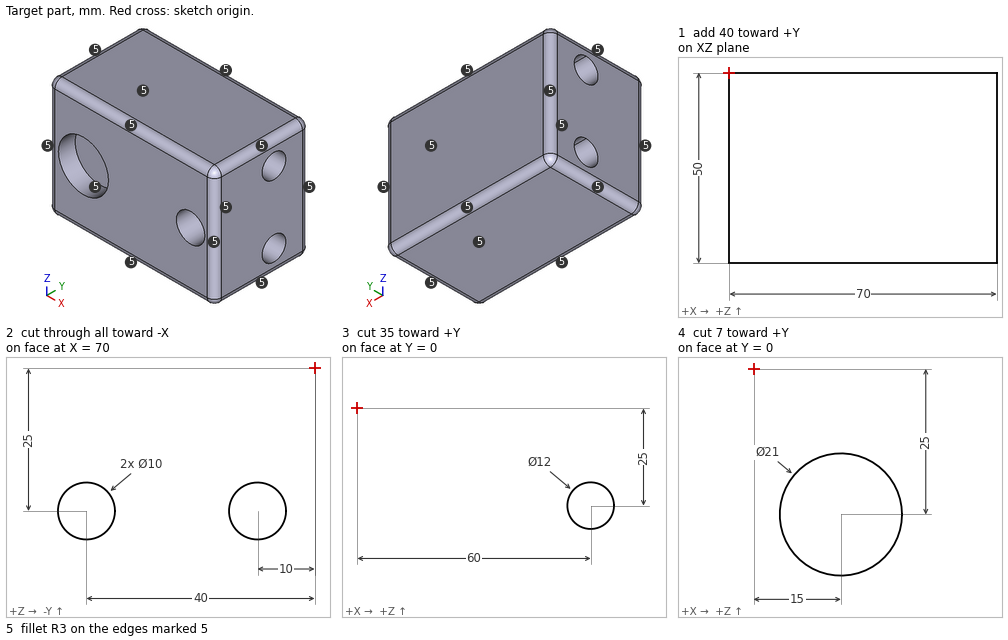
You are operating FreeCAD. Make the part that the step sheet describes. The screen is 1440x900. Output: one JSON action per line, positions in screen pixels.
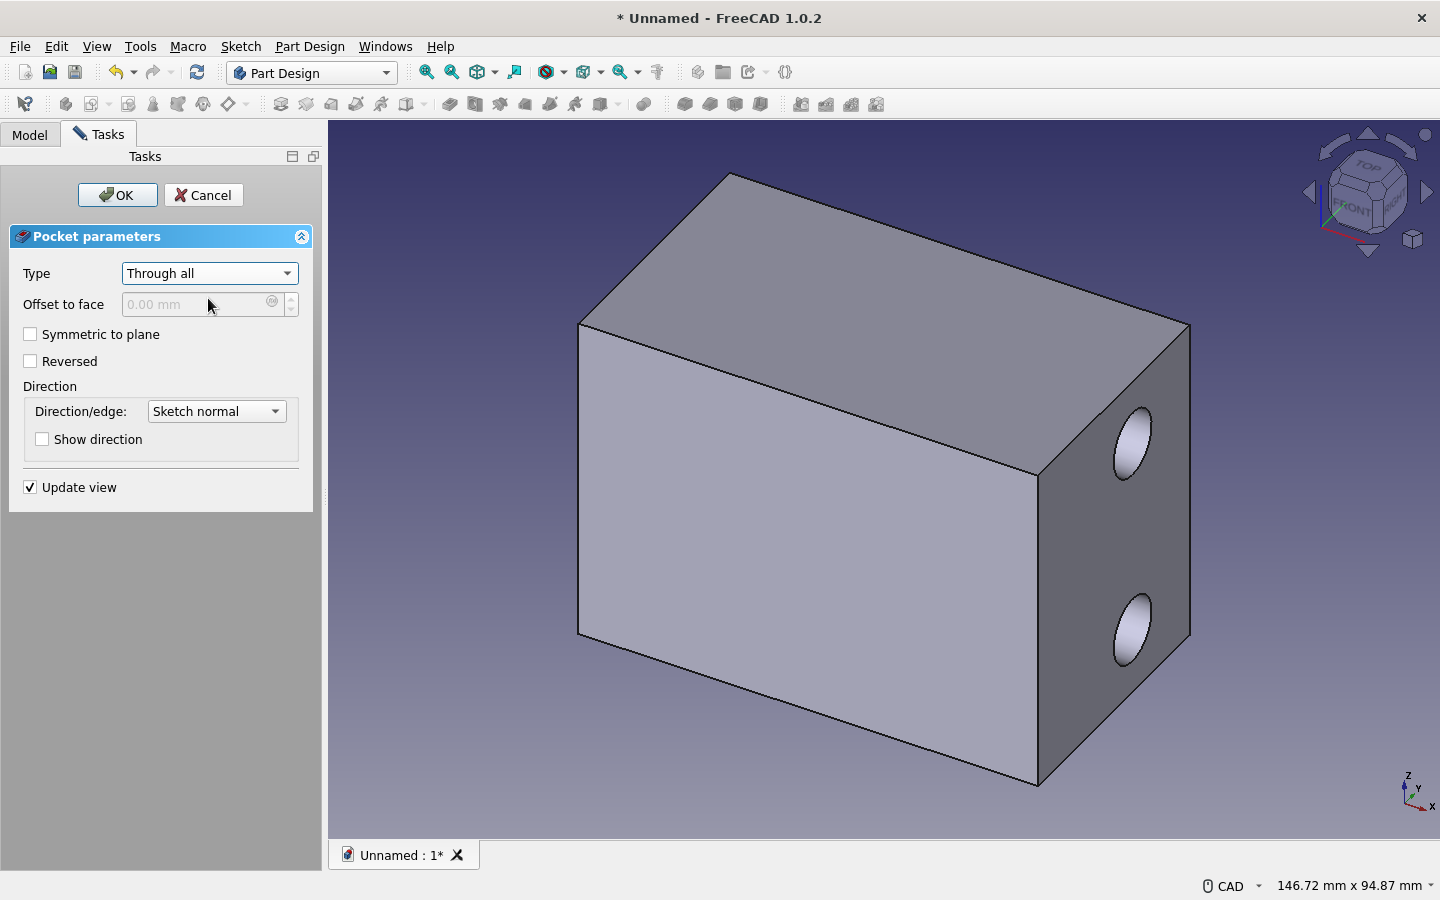
{"action": "left_click", "coordinate": [118, 195]}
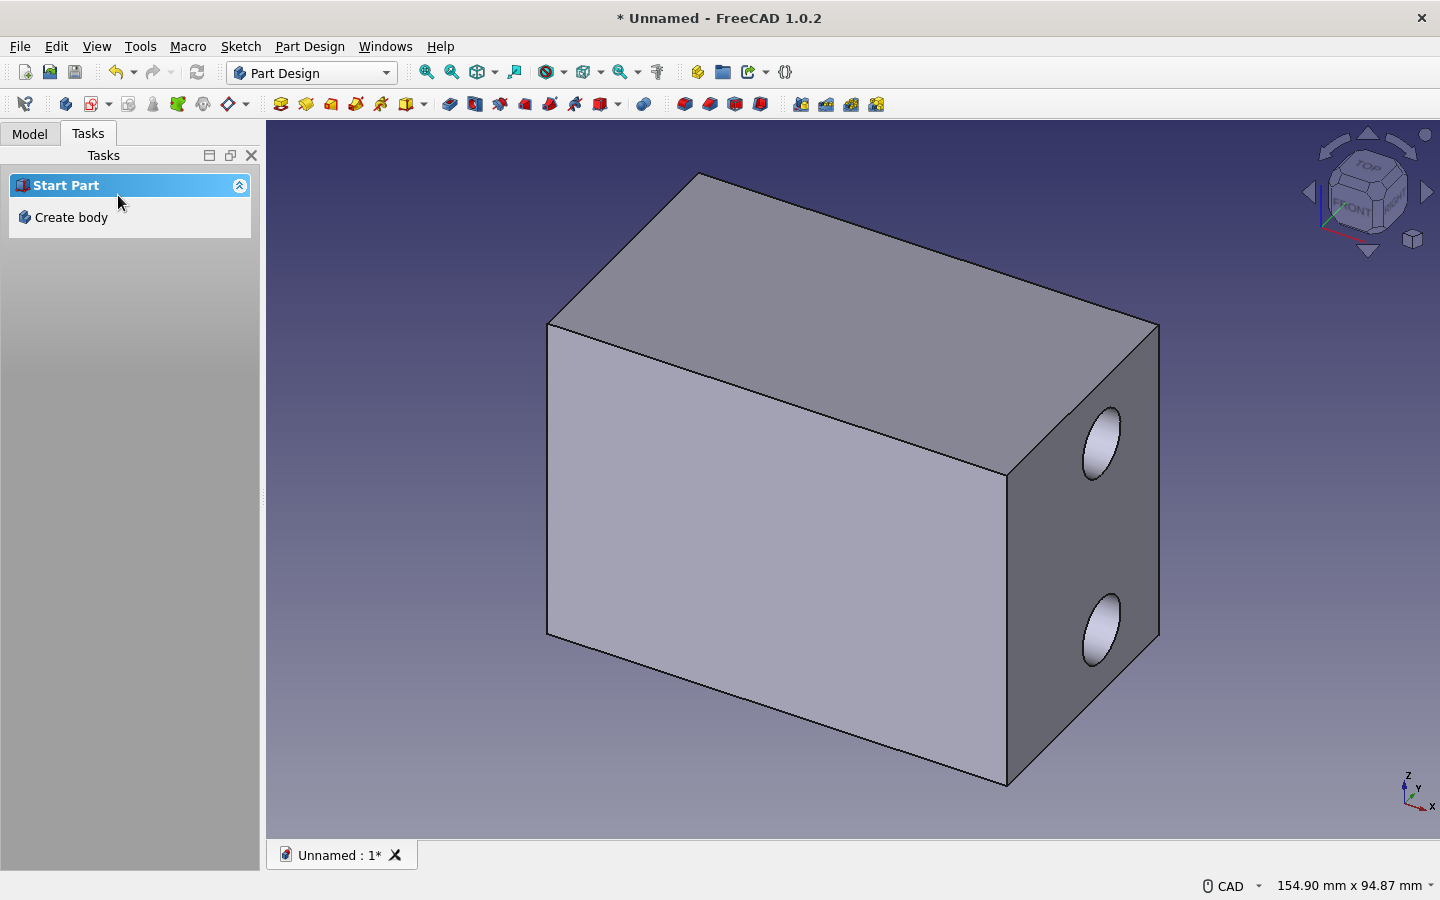
{"action": "left_click", "coordinate": [777, 554]}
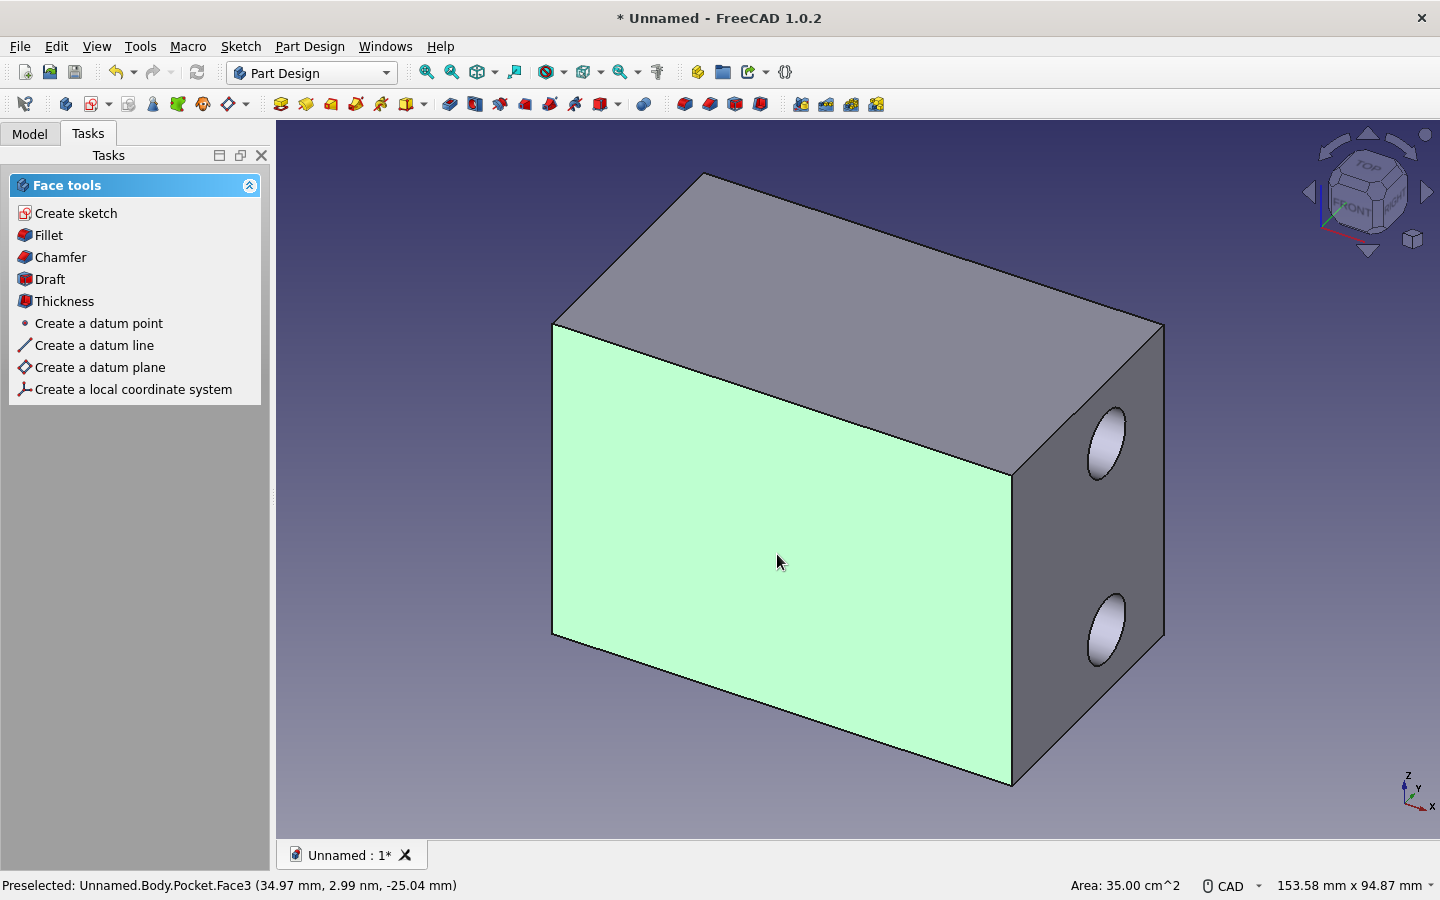
{"action": "left_click", "coordinate": [90, 104]}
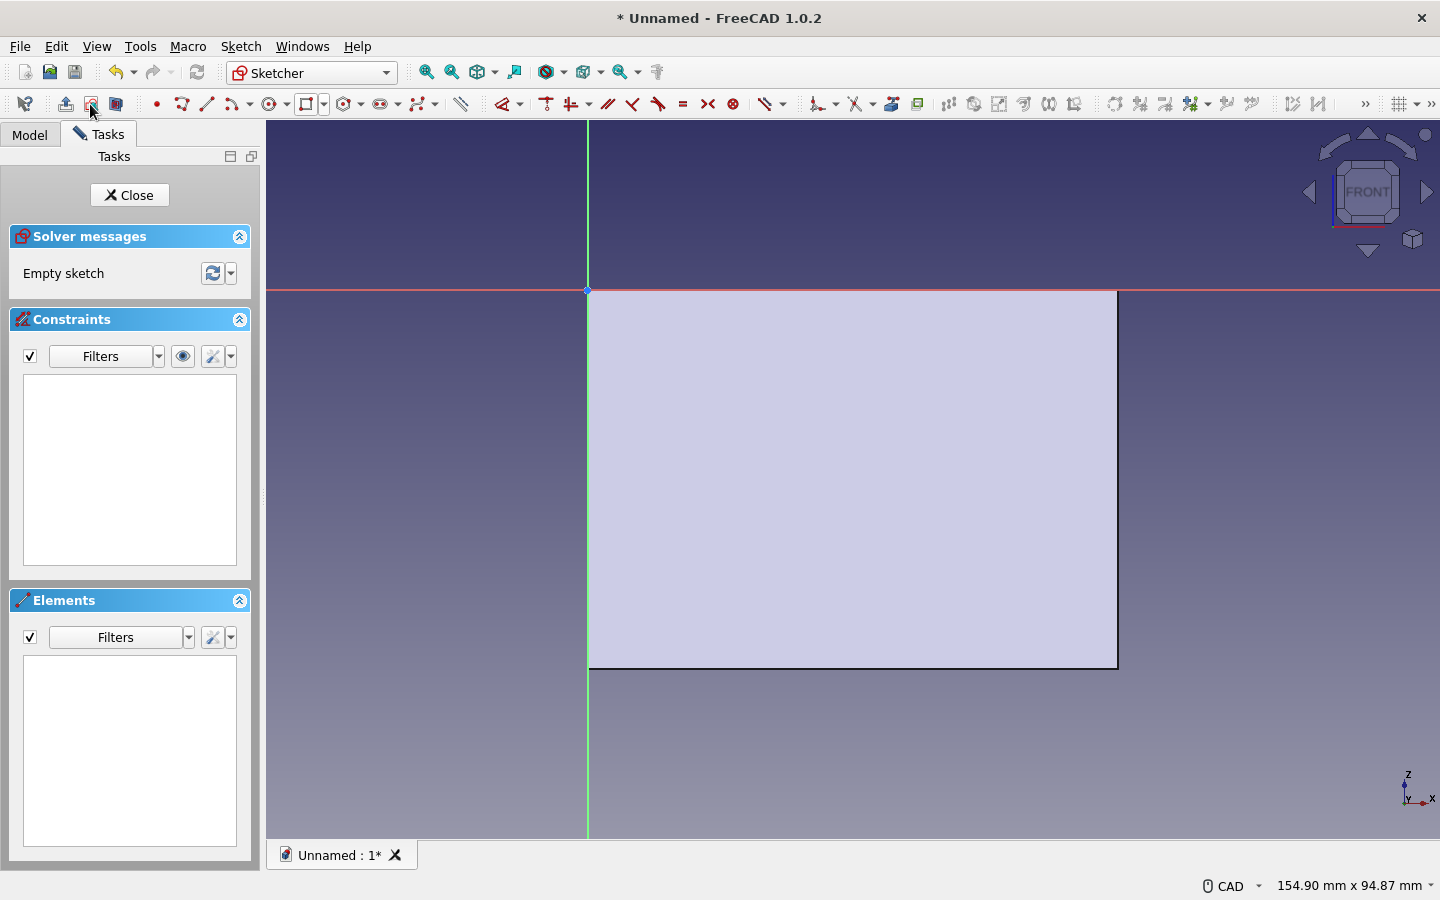
{"action": "scroll", "coordinate": [1108, 479], "scroll_direction": "up", "scroll_amount": 8}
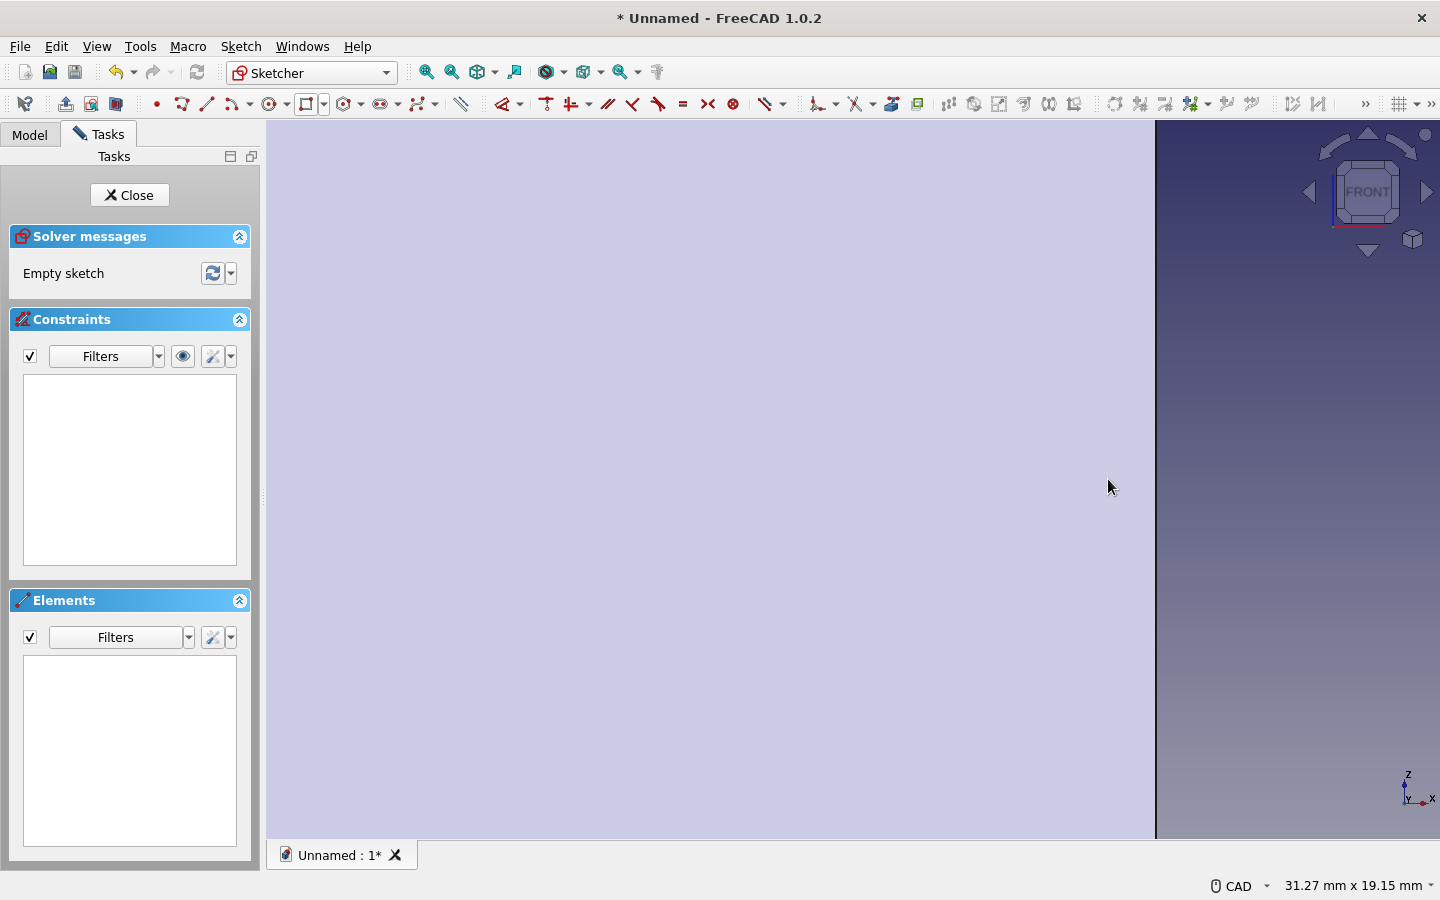
{"action": "key", "text": "g c"}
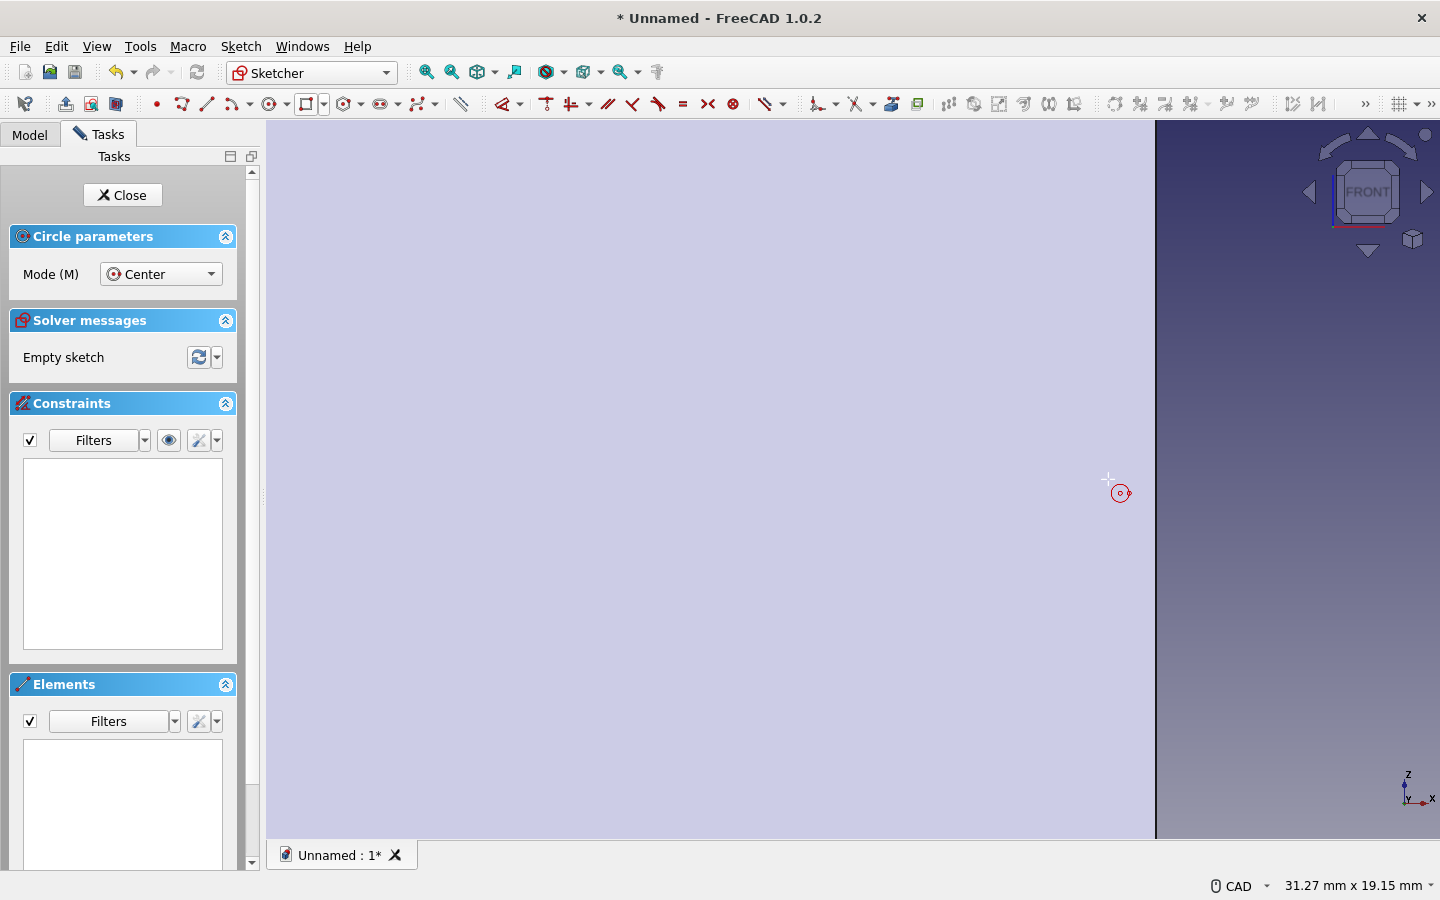
{"action": "left_click", "coordinate": [781, 479]}
{"action": "left_click", "coordinate": [940, 320]}
{"action": "key", "text": "Escape"}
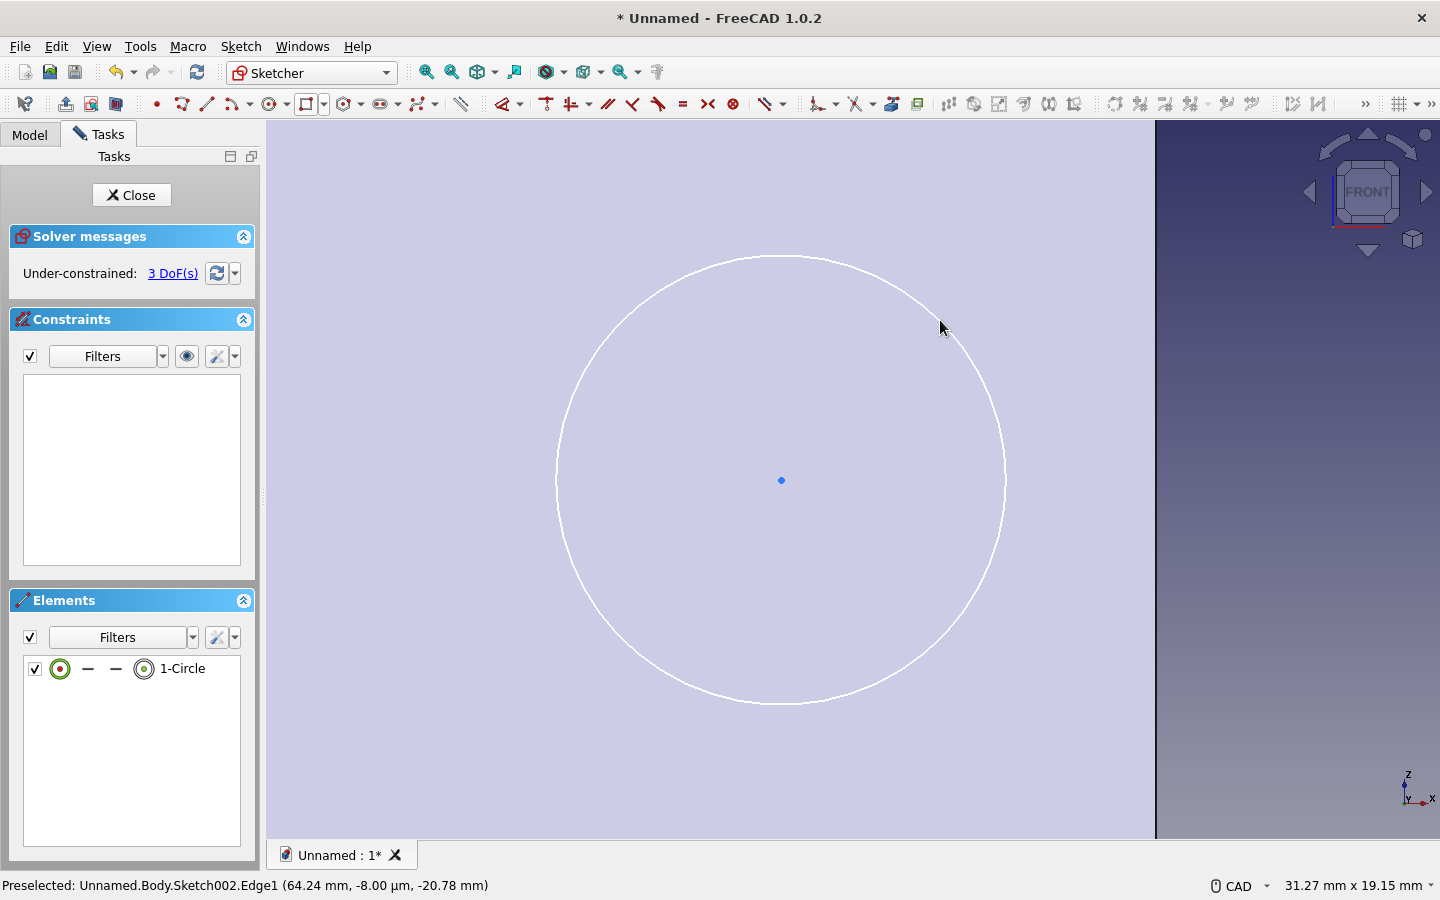
{"action": "left_click", "coordinate": [940, 321]}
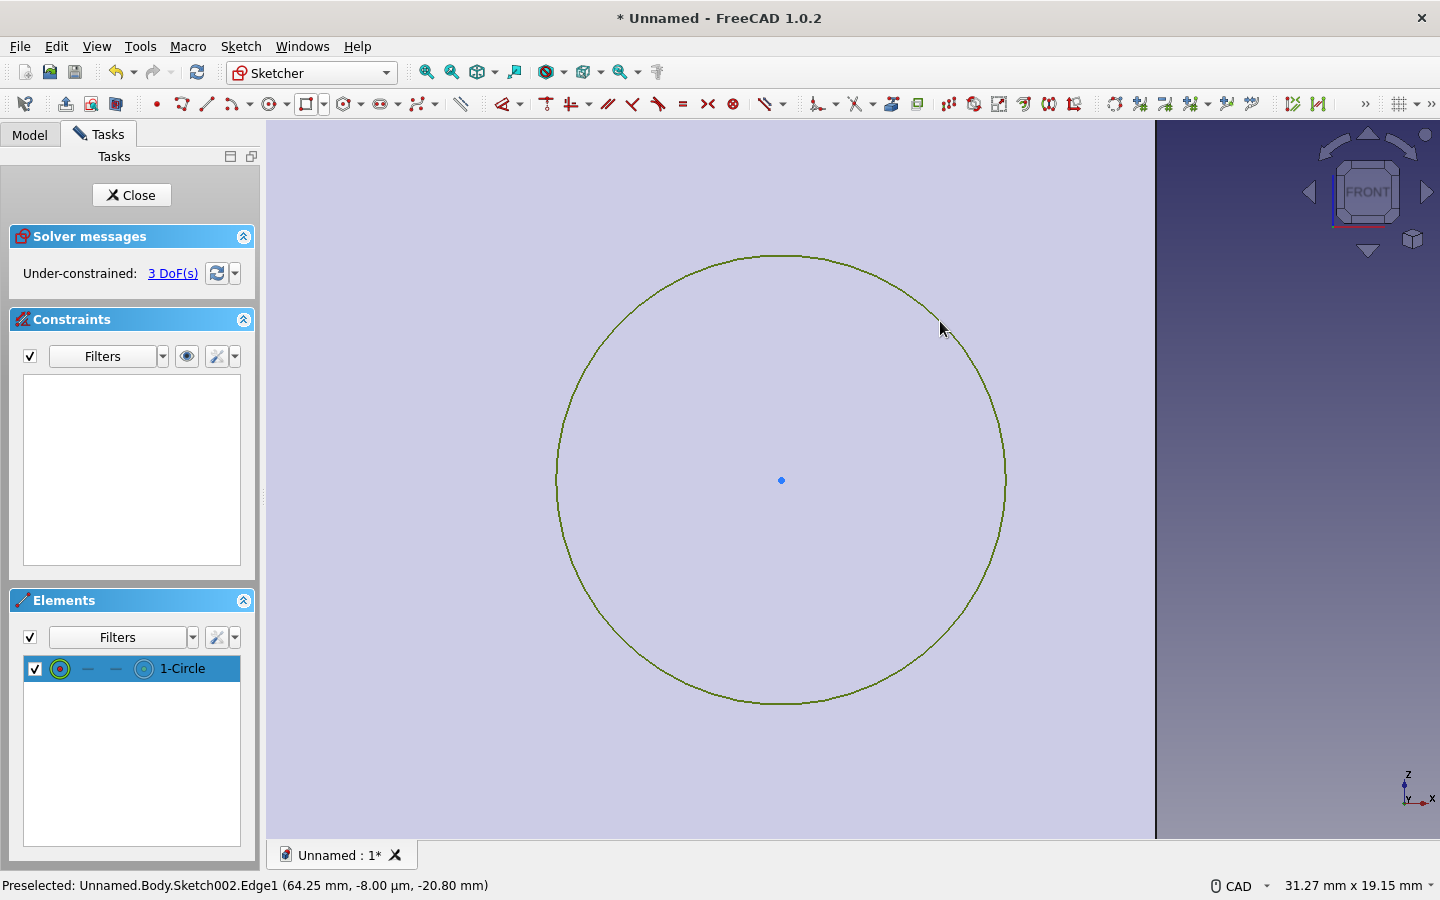
{"action": "key", "text": "k o"}